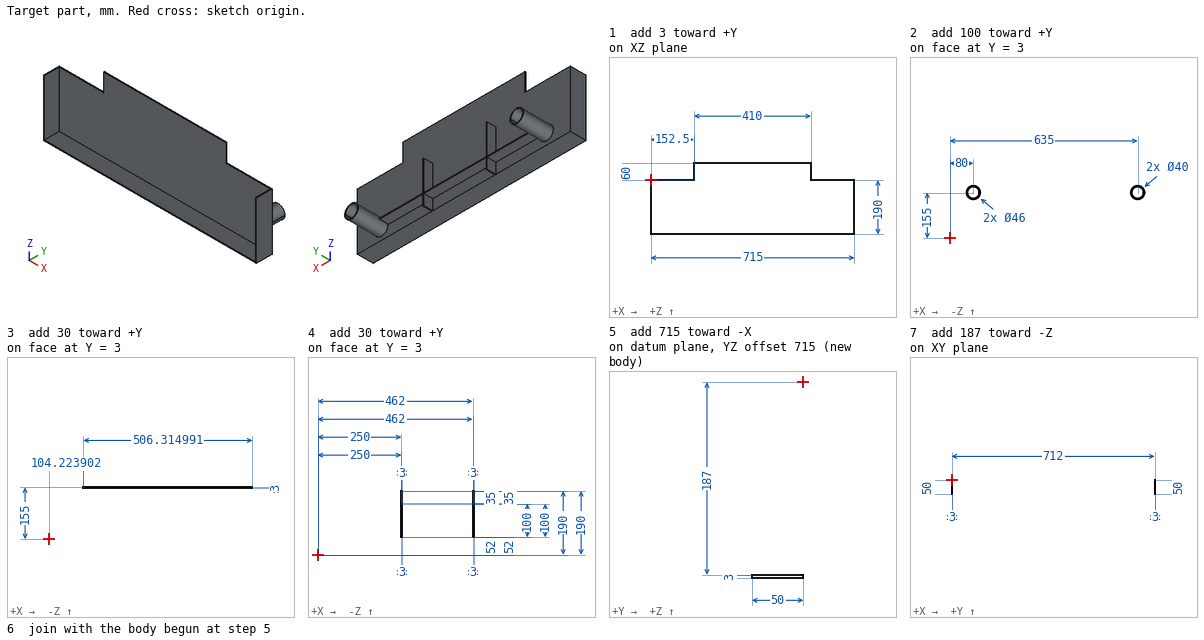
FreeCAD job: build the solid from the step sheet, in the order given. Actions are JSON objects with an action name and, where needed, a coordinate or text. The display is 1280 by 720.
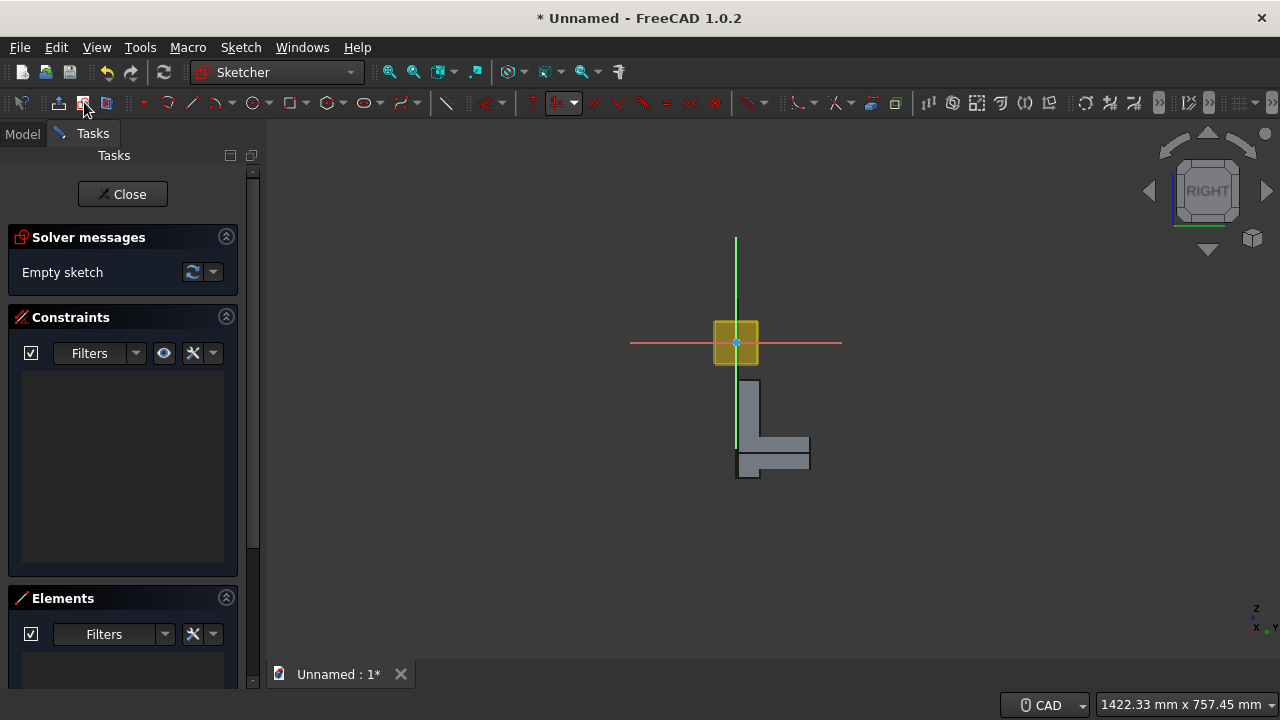
{"action": "scroll", "coordinate": [719, 483], "scroll_direction": "up", "scroll_amount": 14}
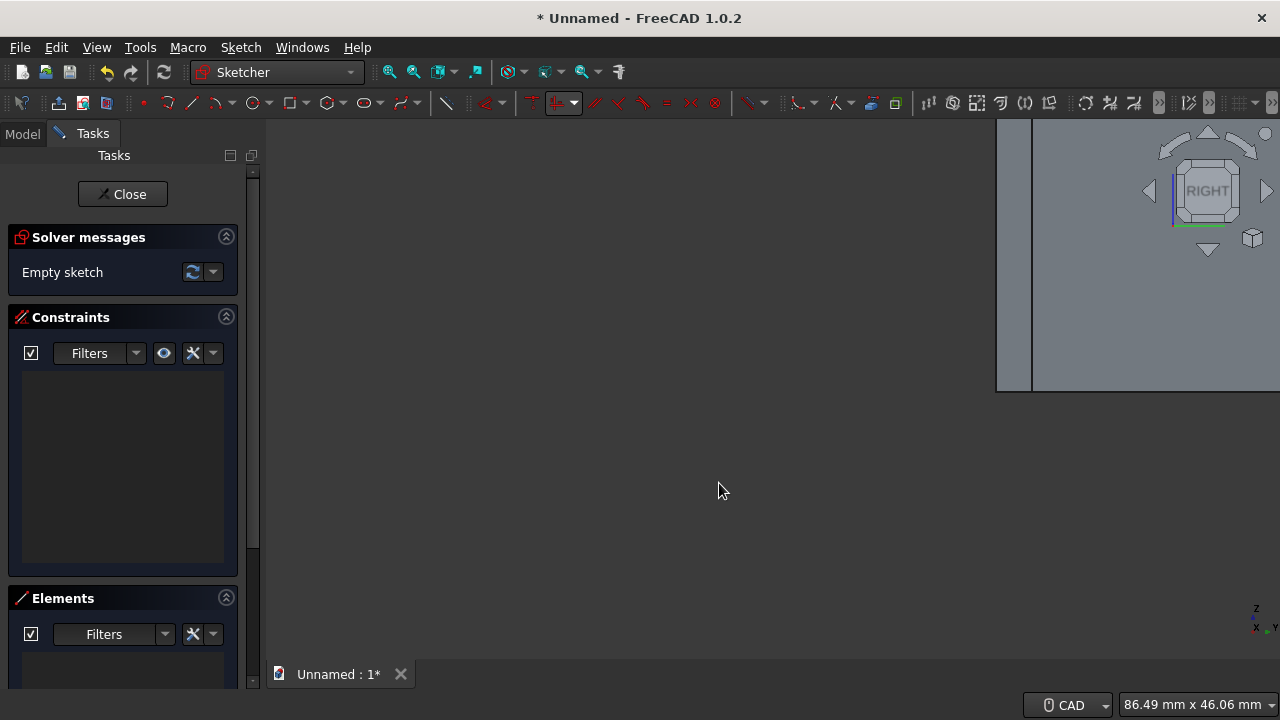
{"action": "left_click", "coordinate": [290, 104]}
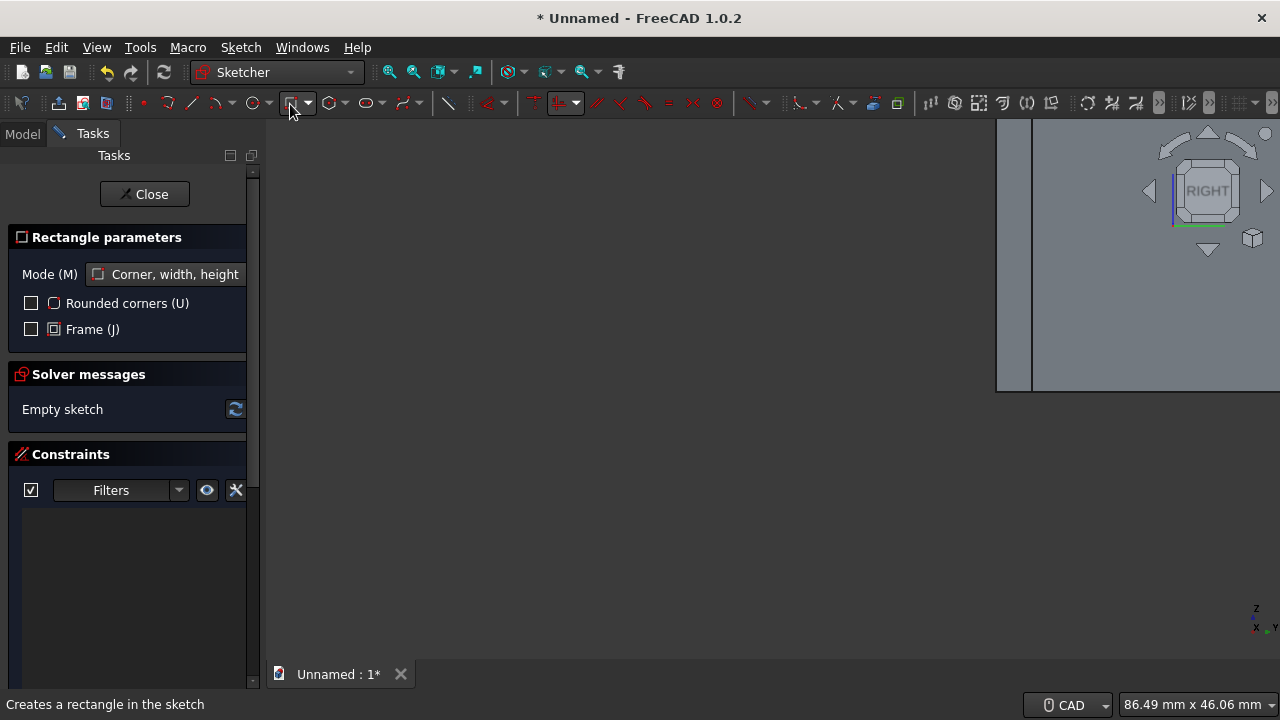
{"action": "left_click", "coordinate": [410, 357]}
{"action": "left_click", "coordinate": [996, 392]}
{"action": "key", "text": "Escape"}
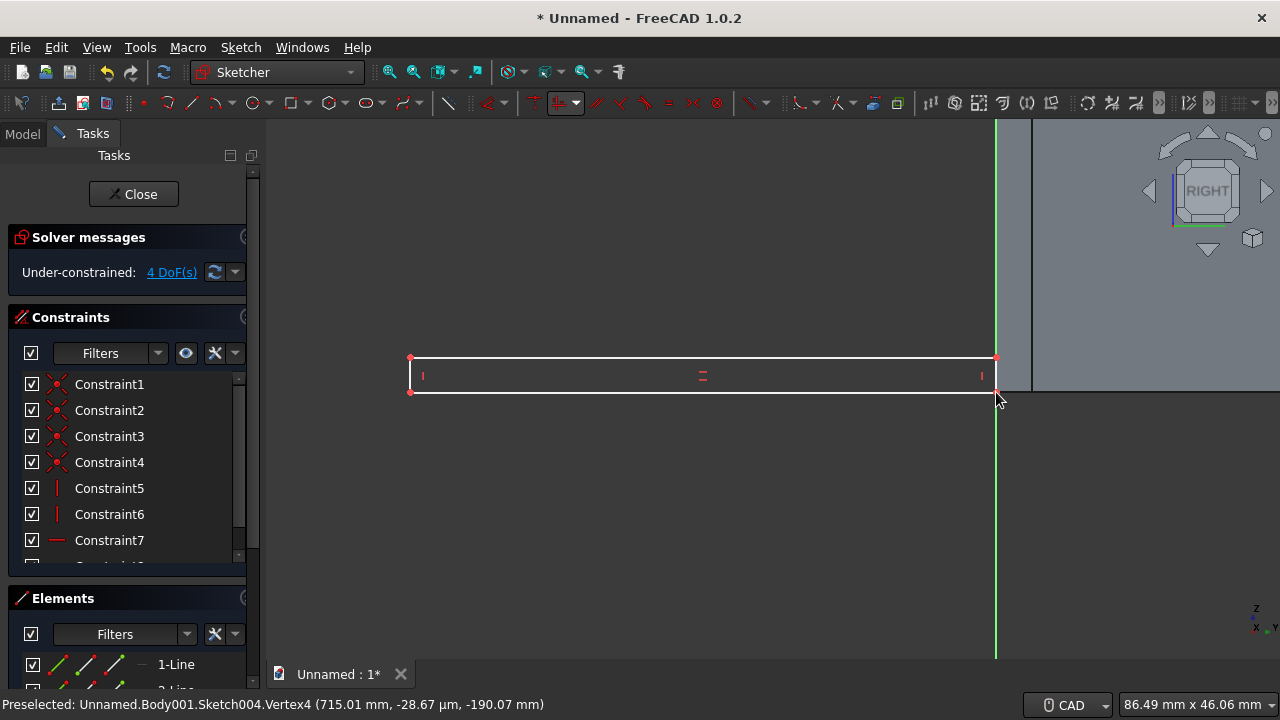
{"action": "left_click", "coordinate": [996, 393]}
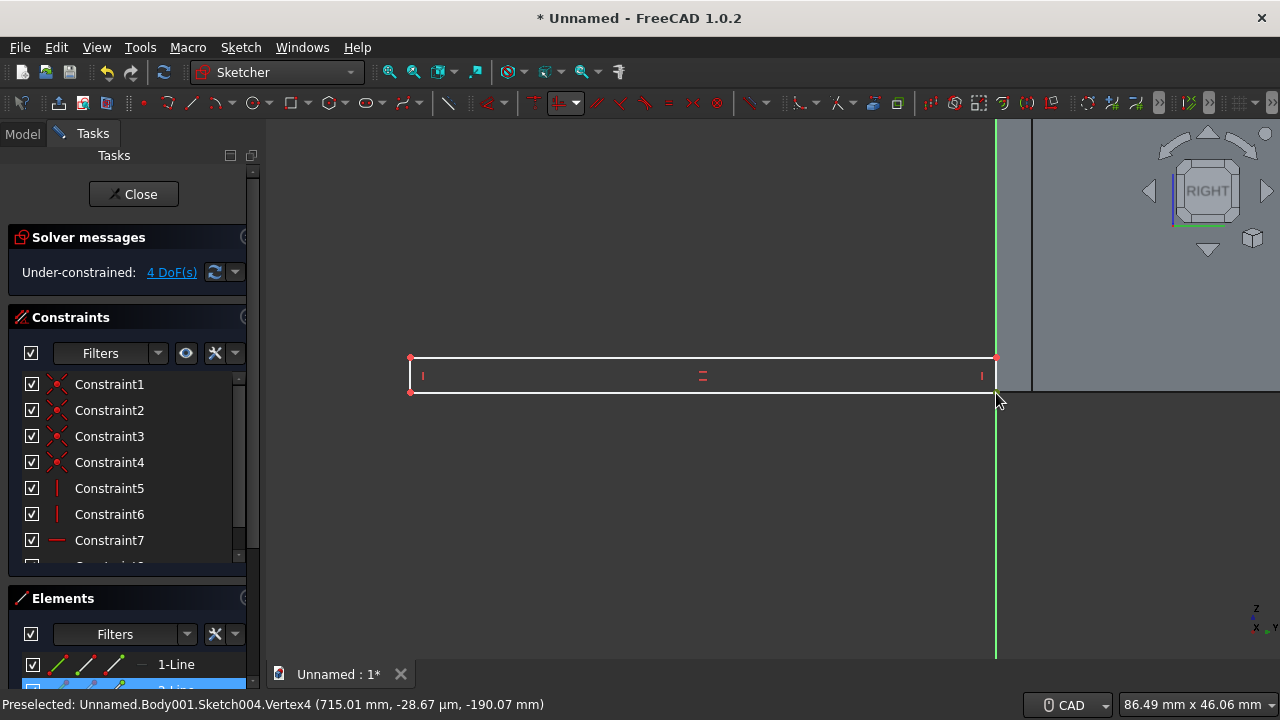
{"action": "left_click", "coordinate": [996, 596]}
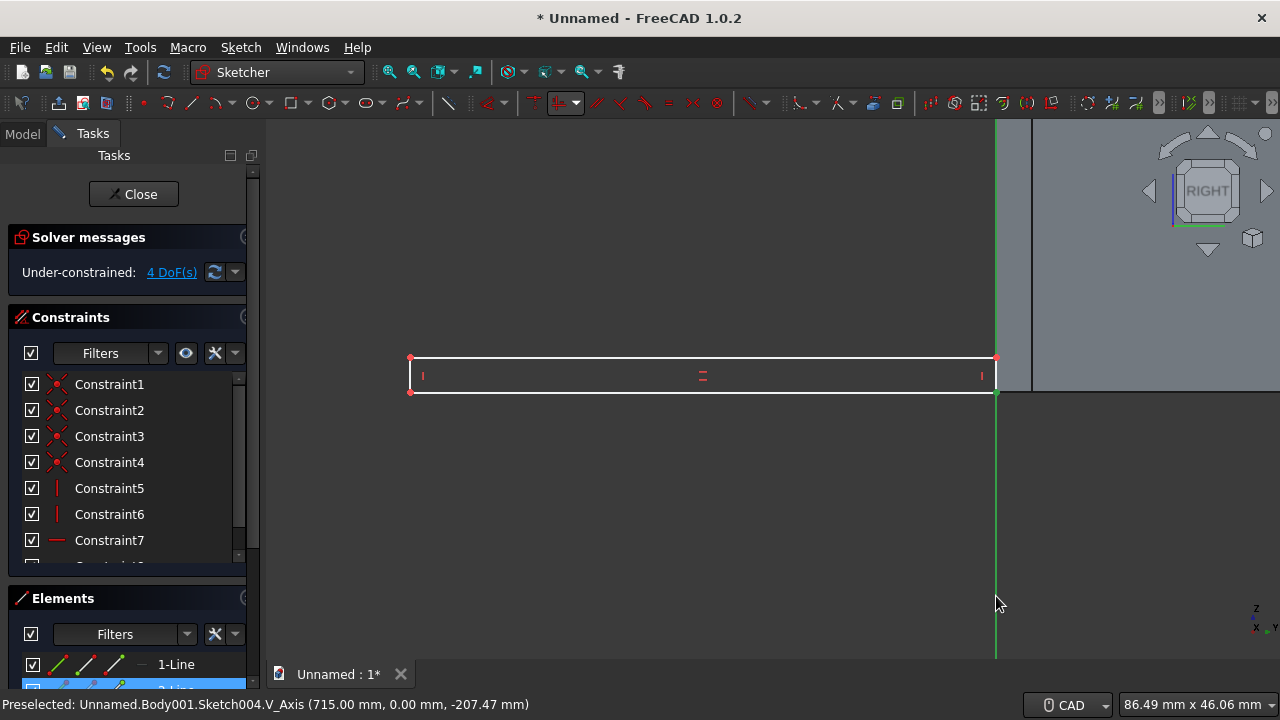
{"action": "left_click", "coordinate": [534, 104]}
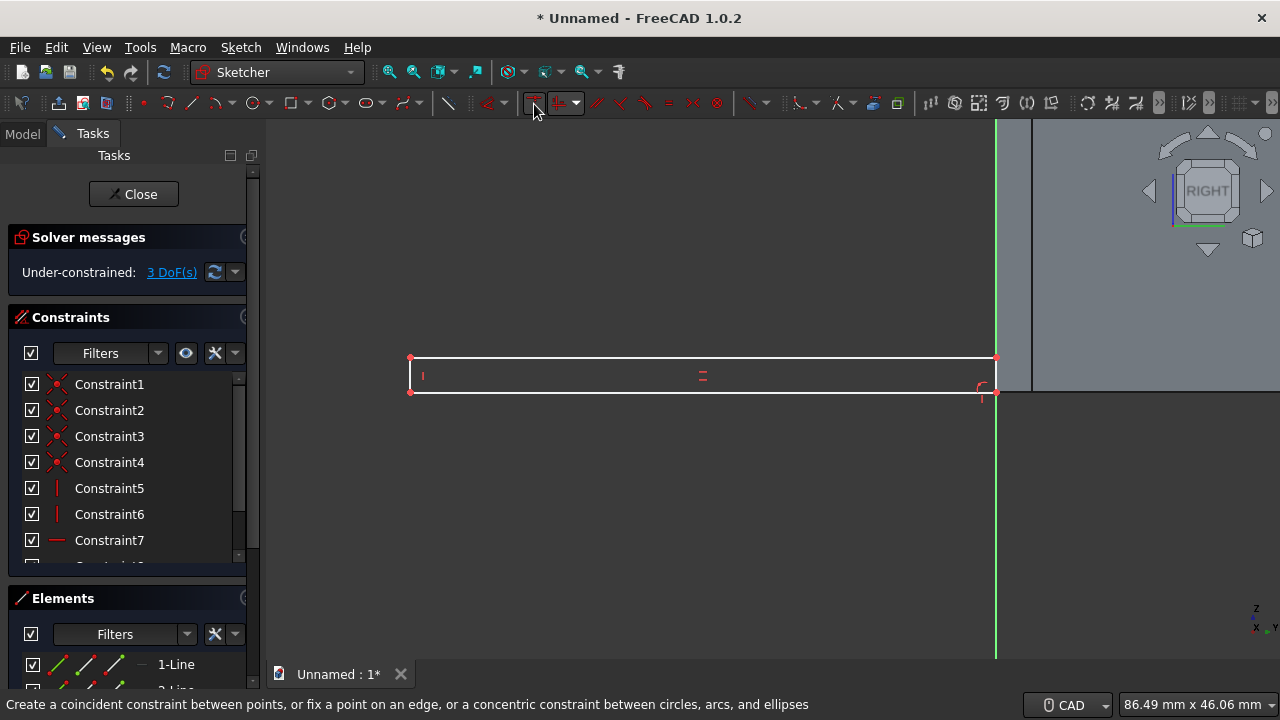
{"action": "left_click", "coordinate": [488, 104]}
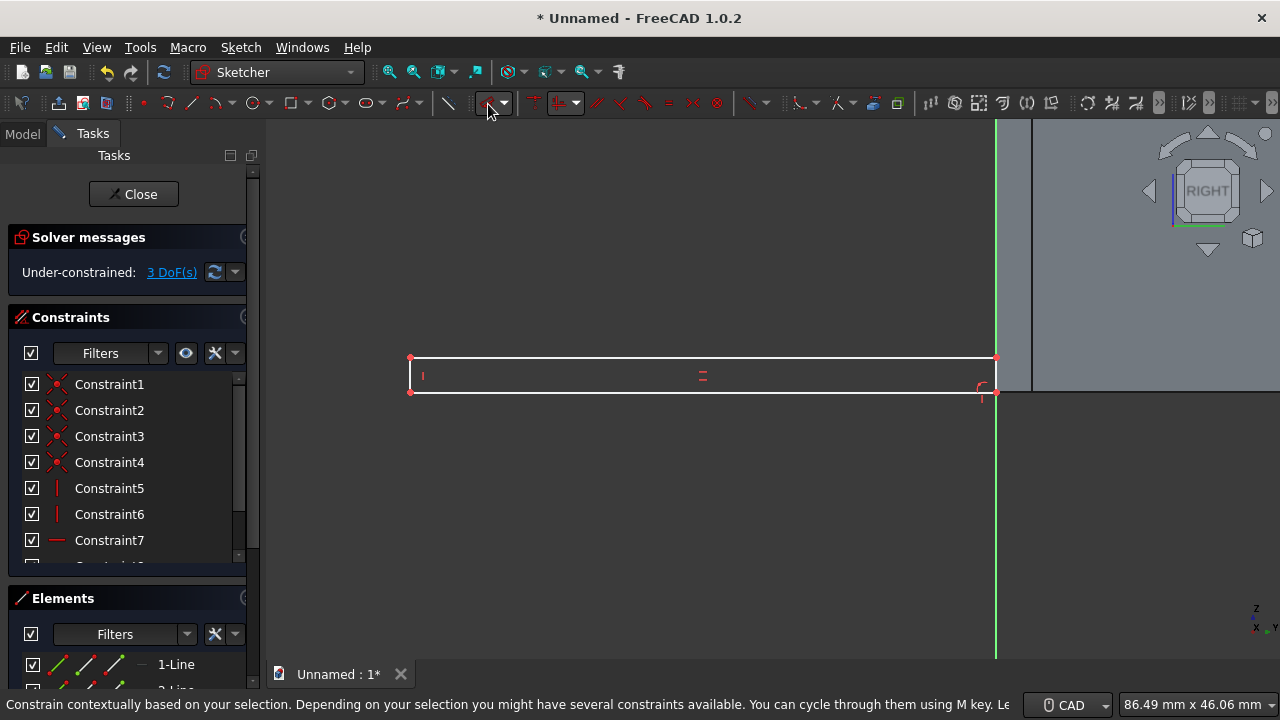
{"action": "scroll", "coordinate": [410, 368], "scroll_direction": "up", "scroll_amount": 2}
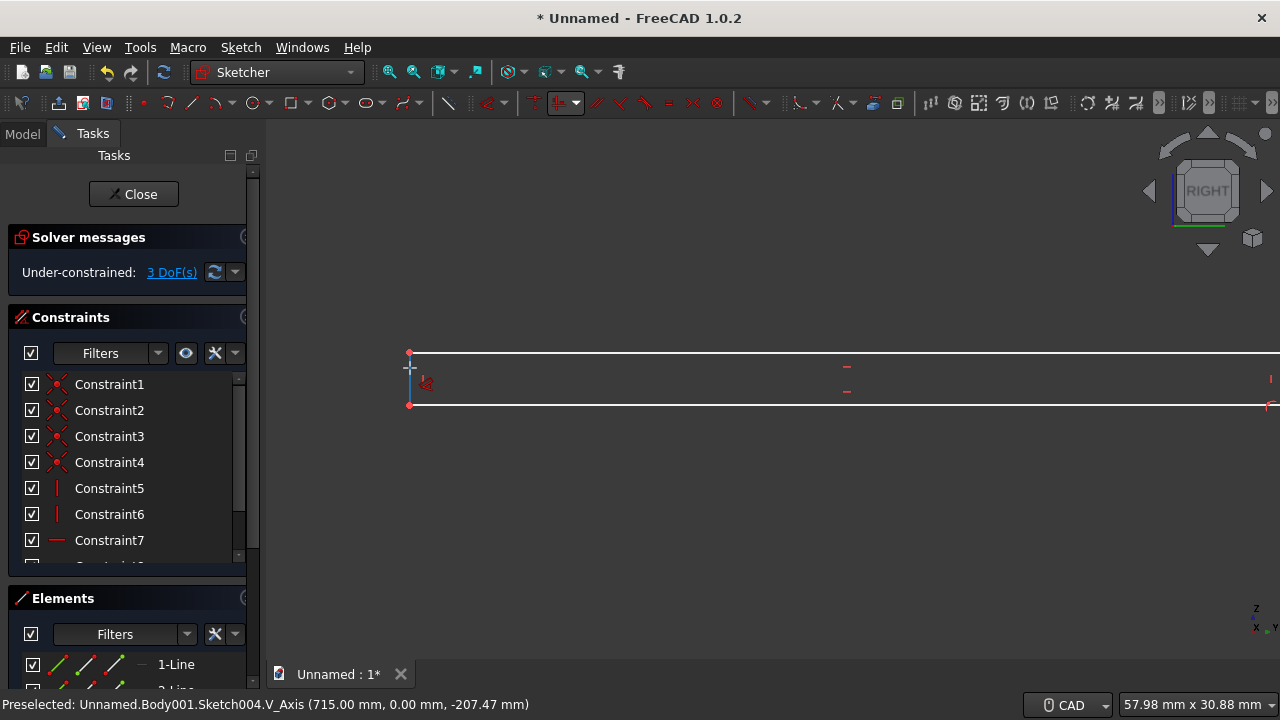
{"action": "left_click", "coordinate": [410, 369]}
{"action": "left_click", "coordinate": [376, 379]}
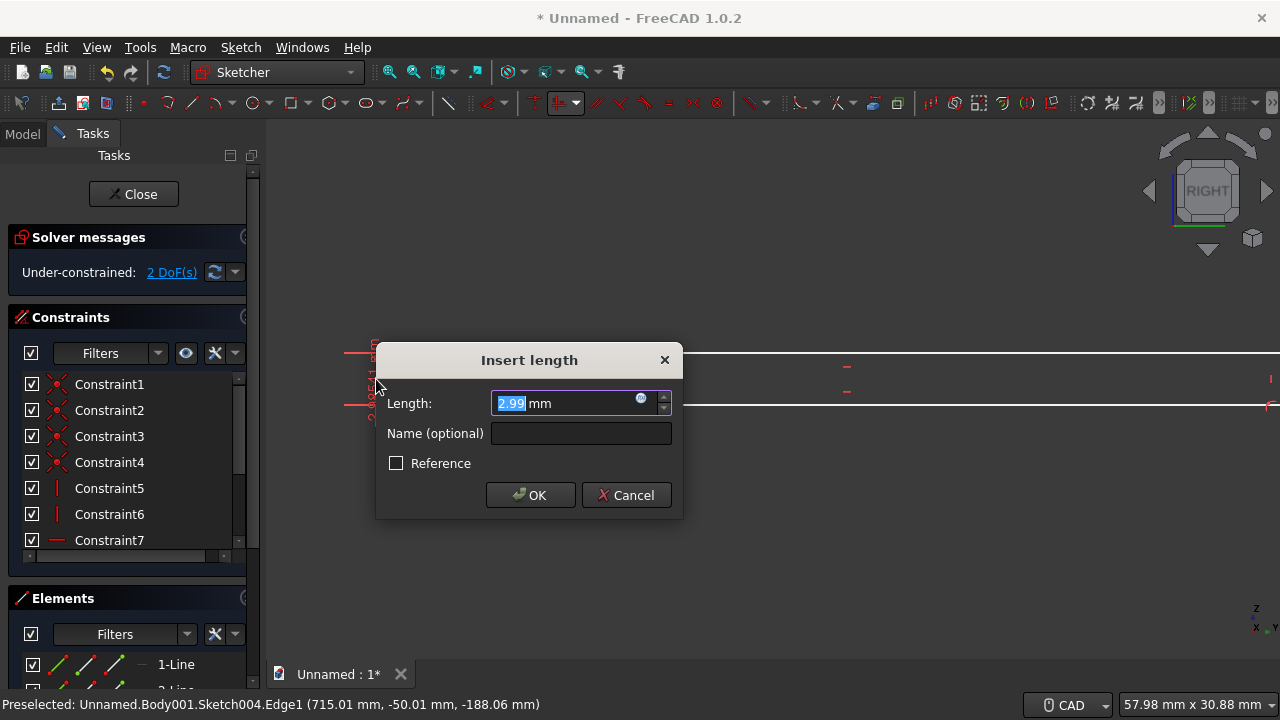
{"action": "type", "text": "3"}
{"action": "key", "text": "Return"}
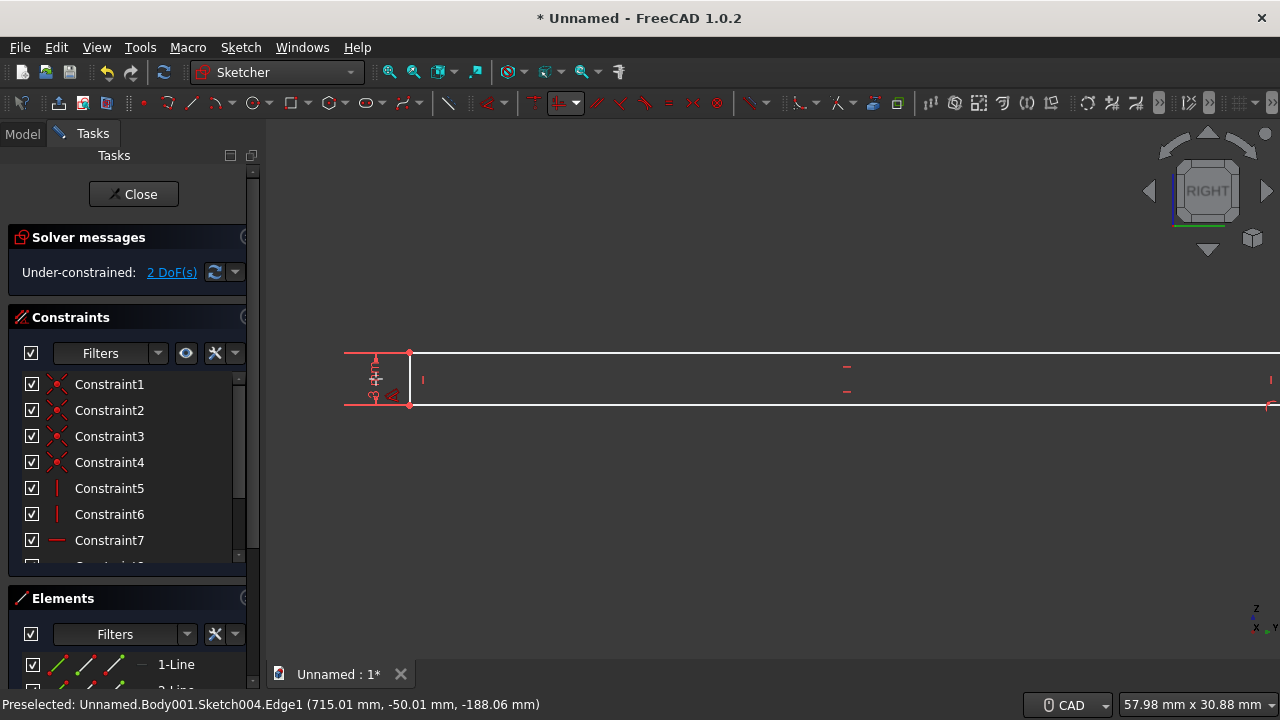
{"action": "left_click", "coordinate": [672, 405]}
{"action": "left_click", "coordinate": [762, 439]}